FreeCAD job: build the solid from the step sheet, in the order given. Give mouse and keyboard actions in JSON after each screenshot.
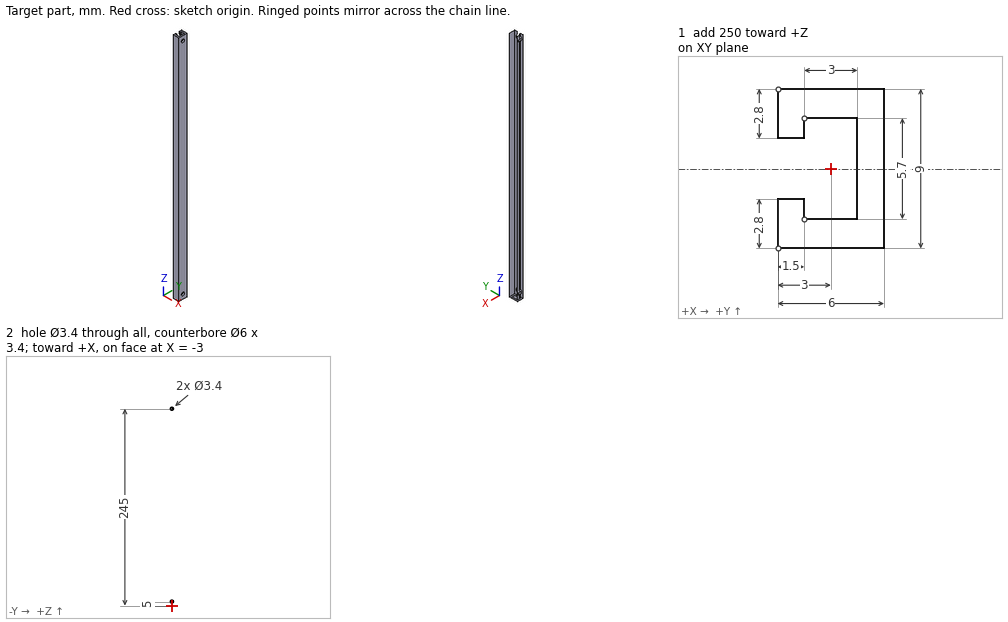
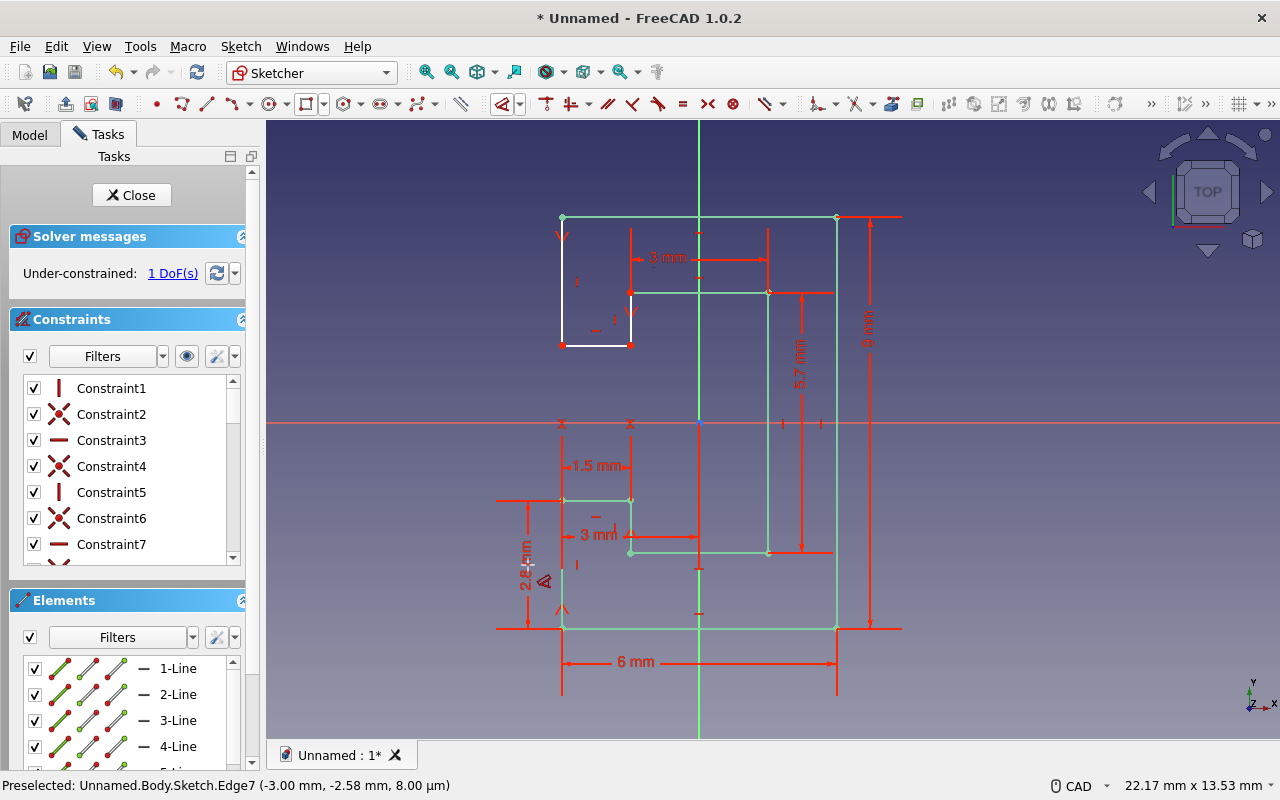
{"action": "left_click", "coordinate": [562, 256]}
{"action": "left_click", "coordinate": [528, 282]}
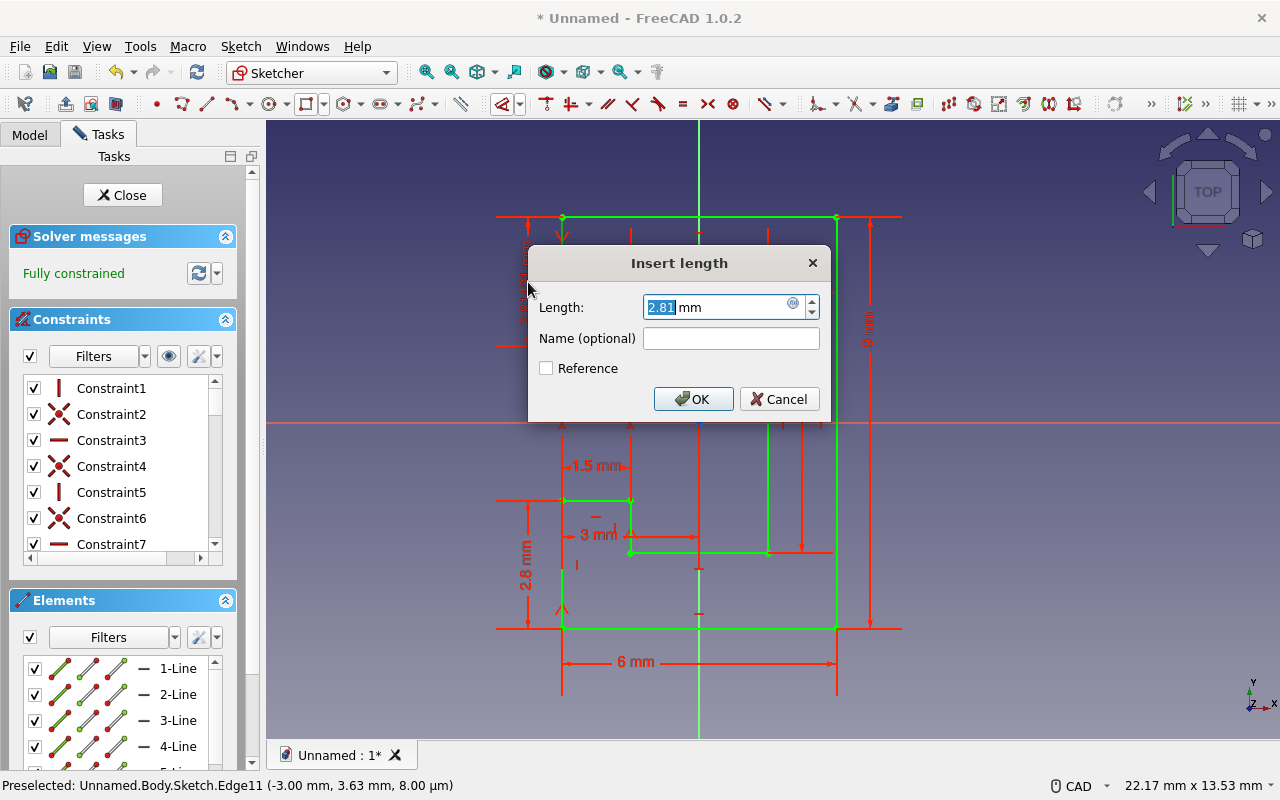
{"action": "type", "text": "2.8"}
{"action": "key", "text": "Return"}
{"action": "key", "text": "Escape"}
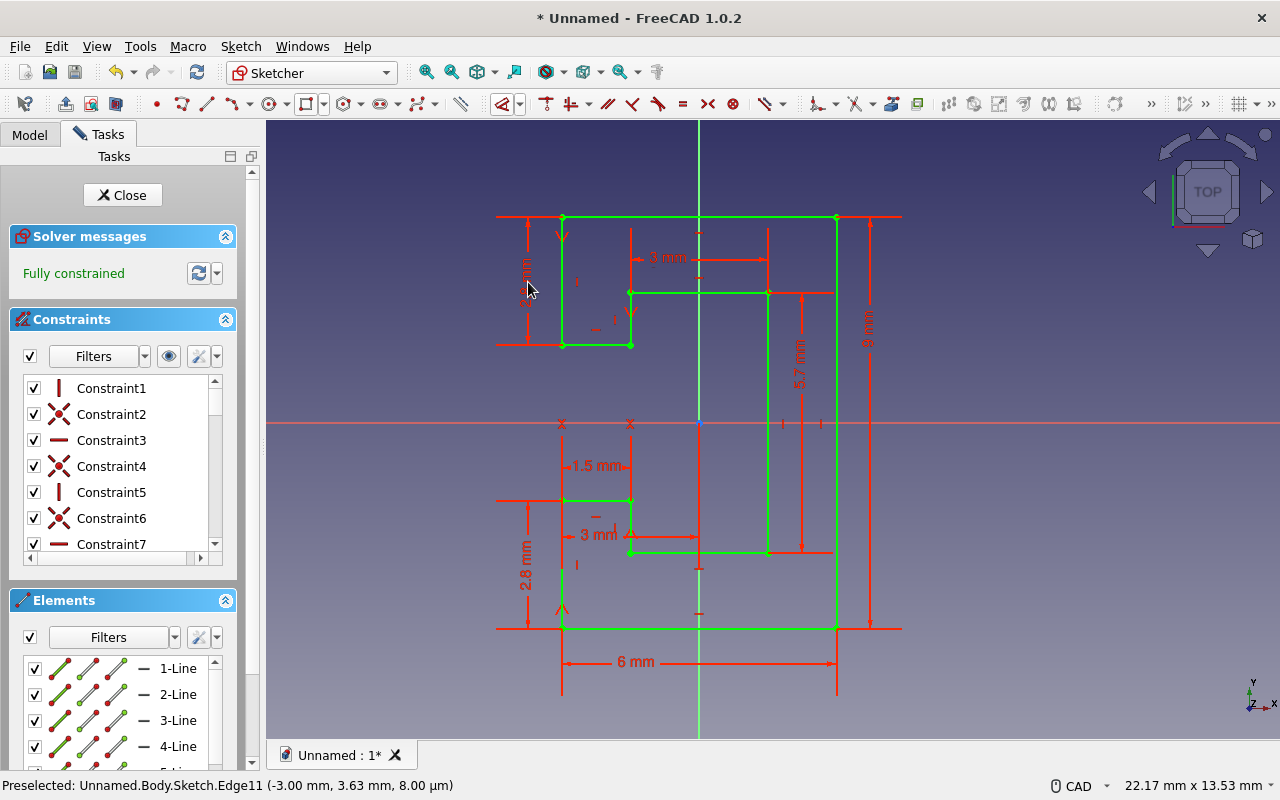
{"action": "left_click", "coordinate": [123, 195]}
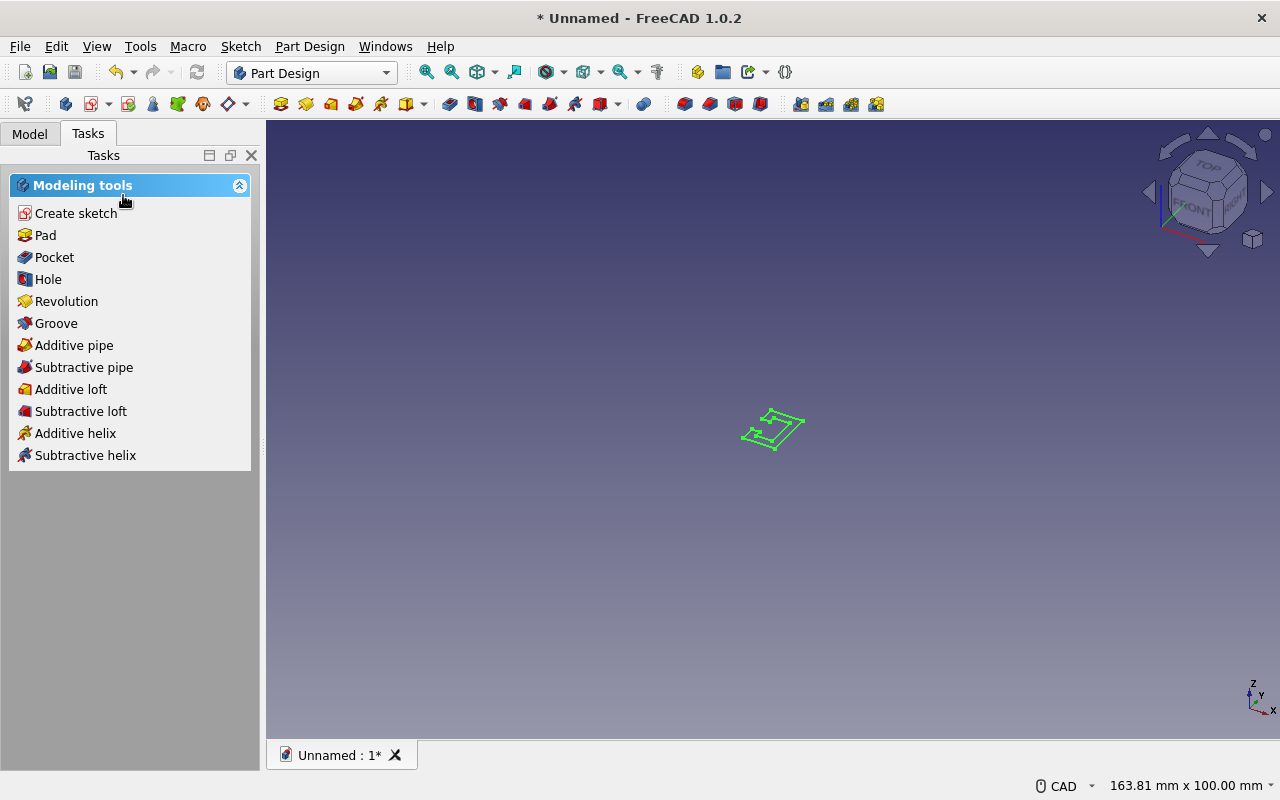
{"action": "left_click", "coordinate": [281, 104]}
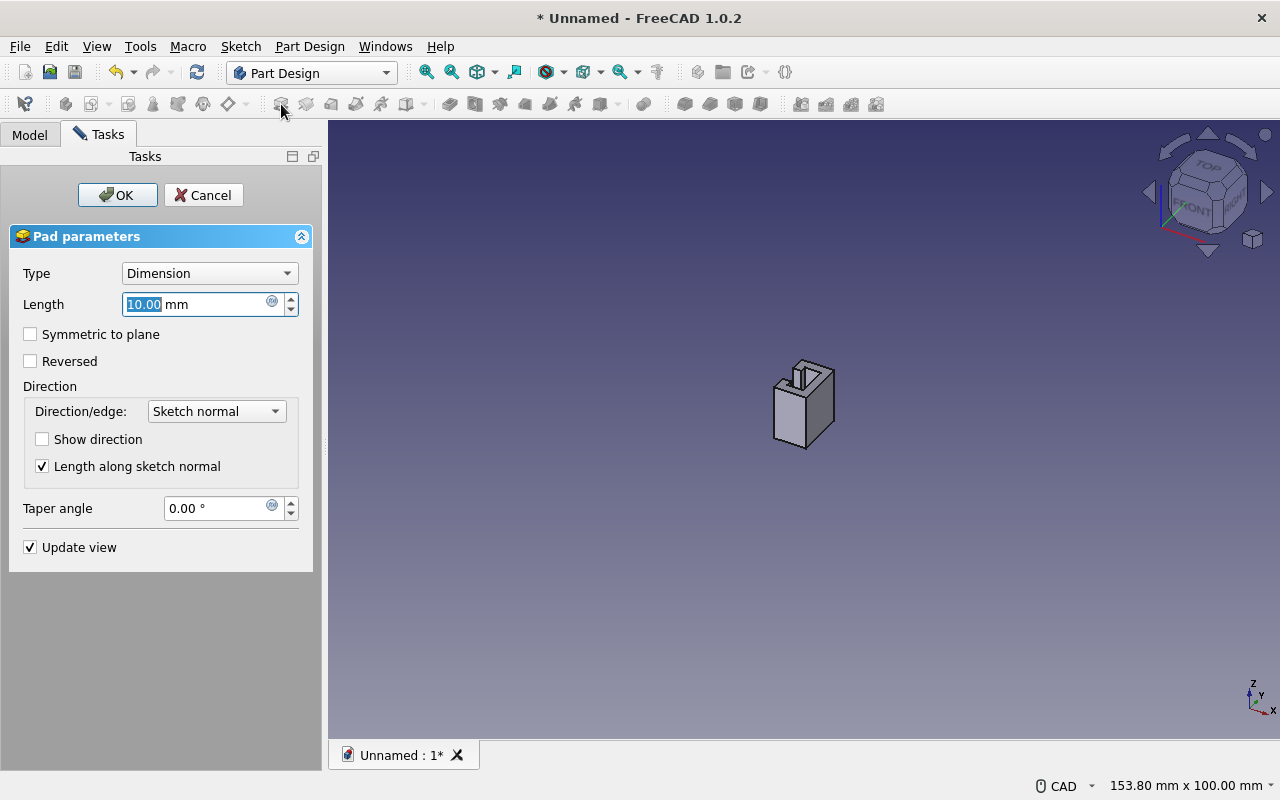
{"action": "type", "text": "250"}
{"action": "key", "text": "Tab"}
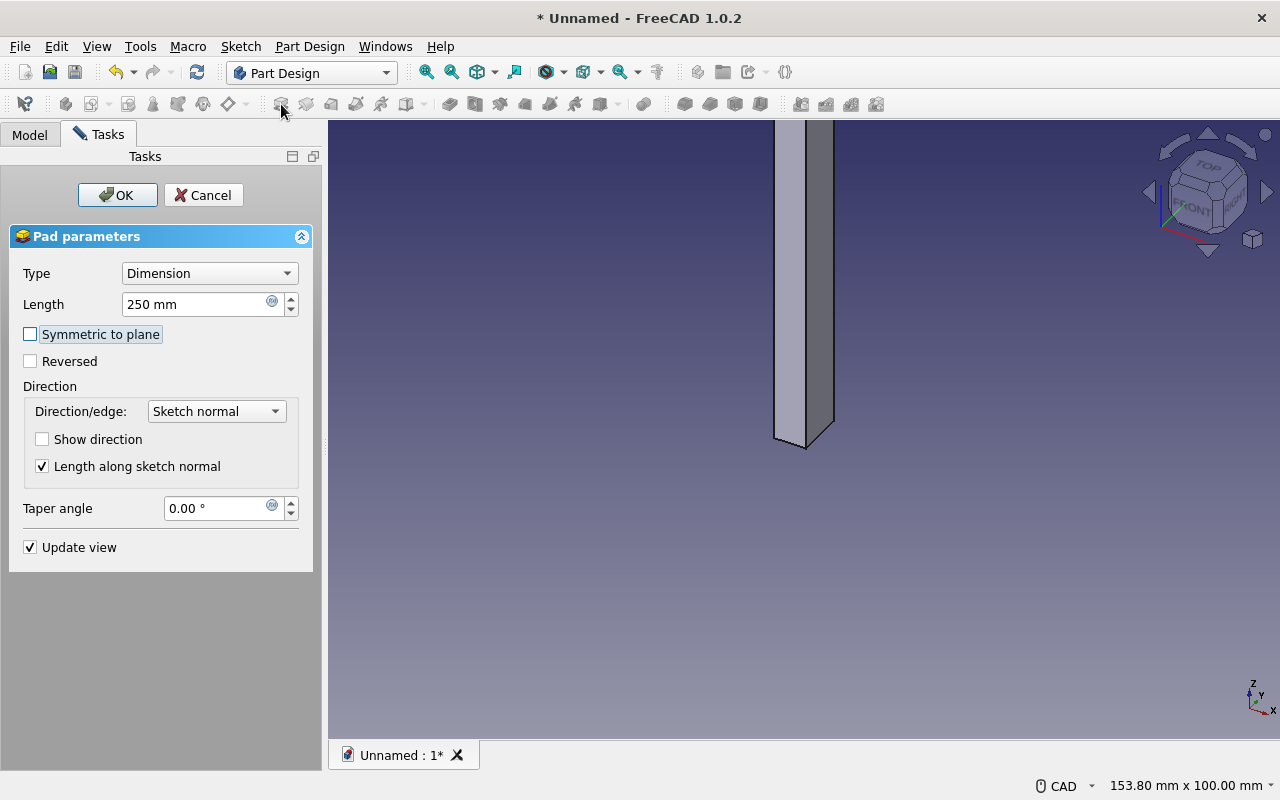
{"action": "left_click", "coordinate": [118, 195]}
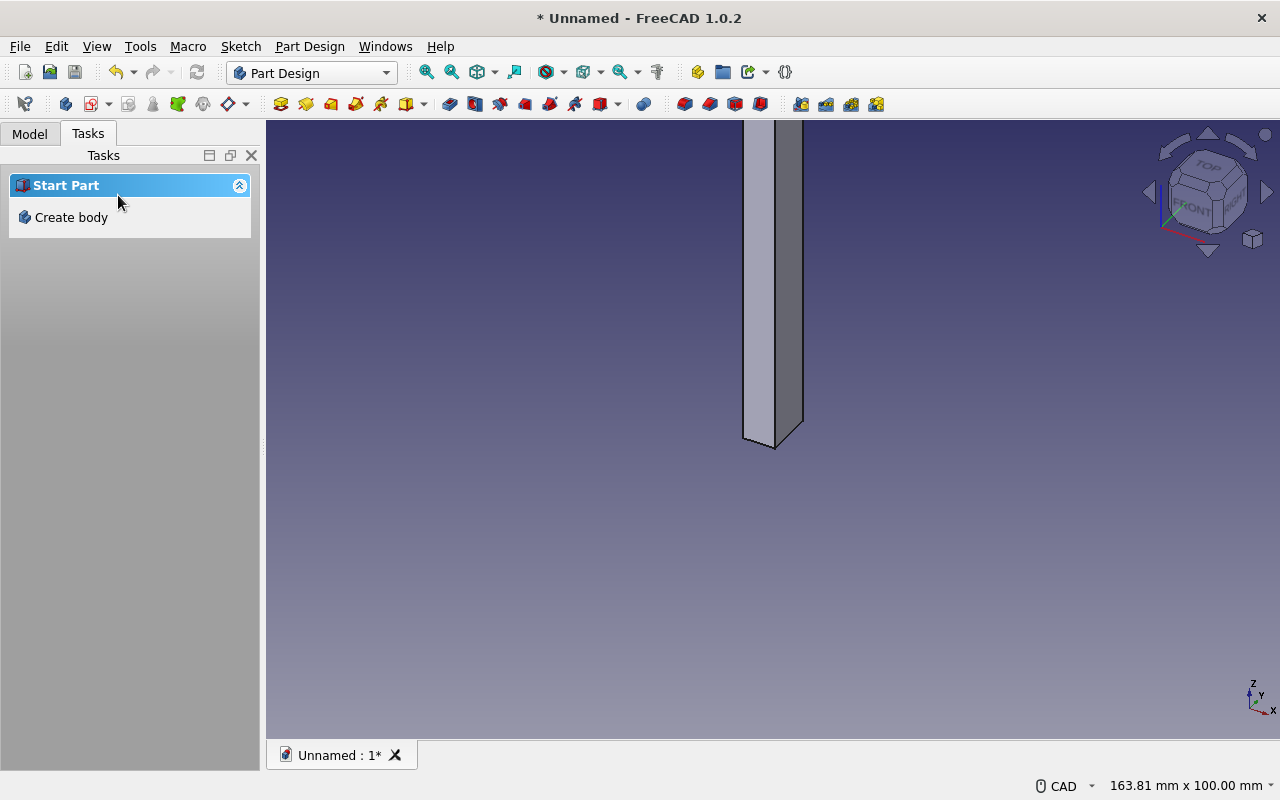
{"action": "key", "text": "v f"}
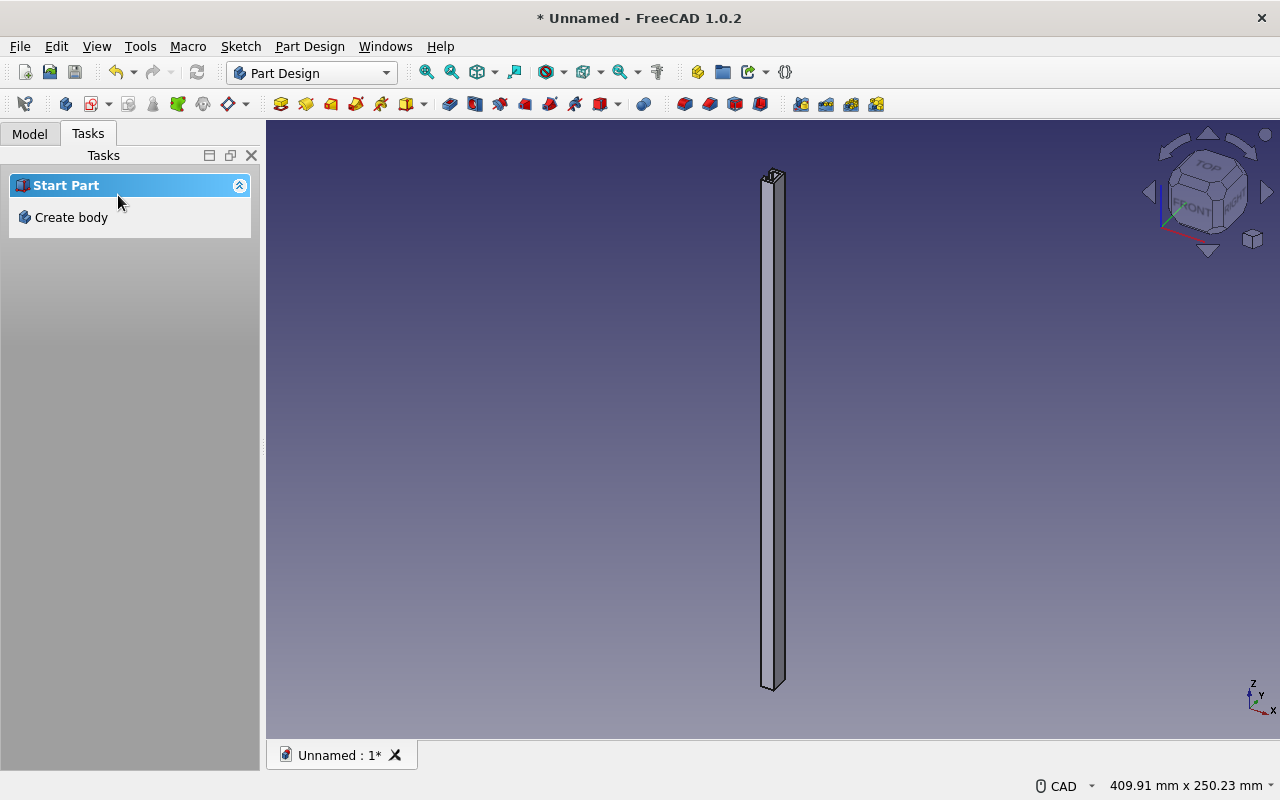
{"action": "key", "text": "6"}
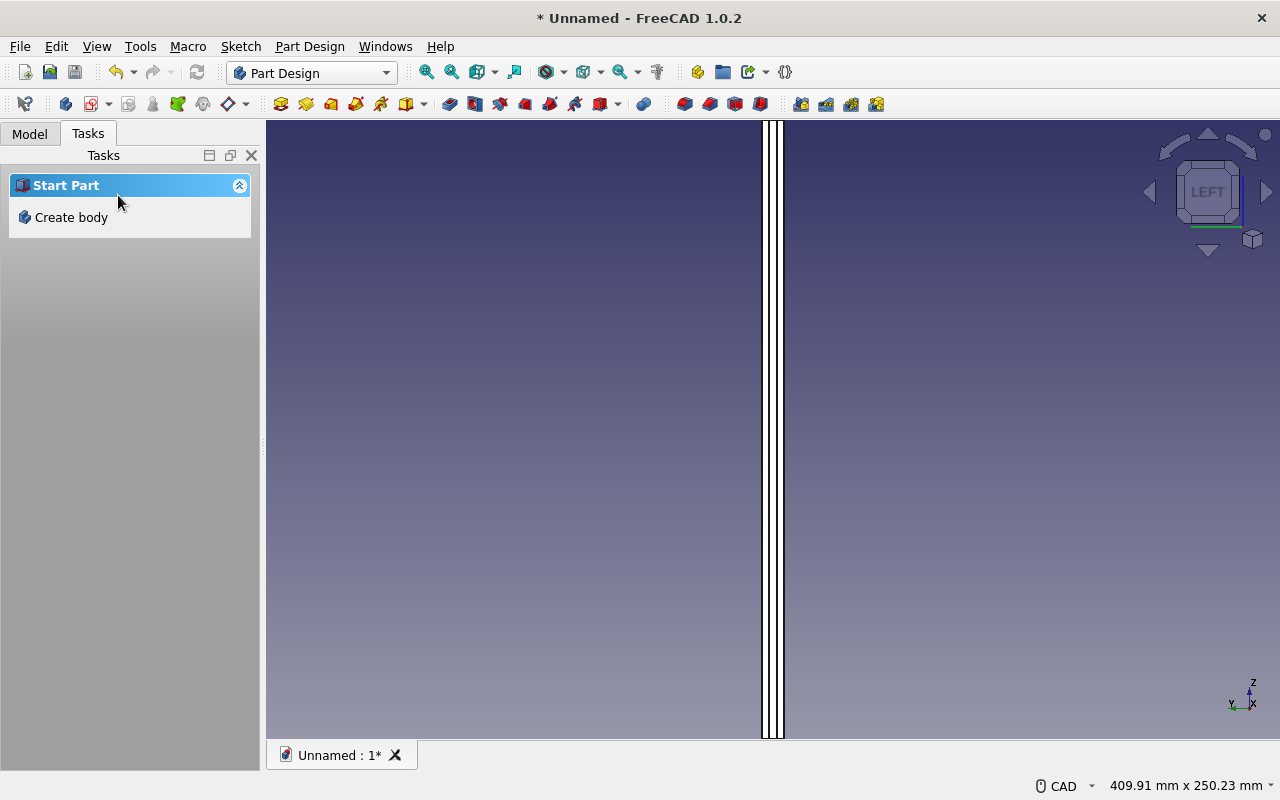
{"action": "left_click", "coordinate": [427, 72]}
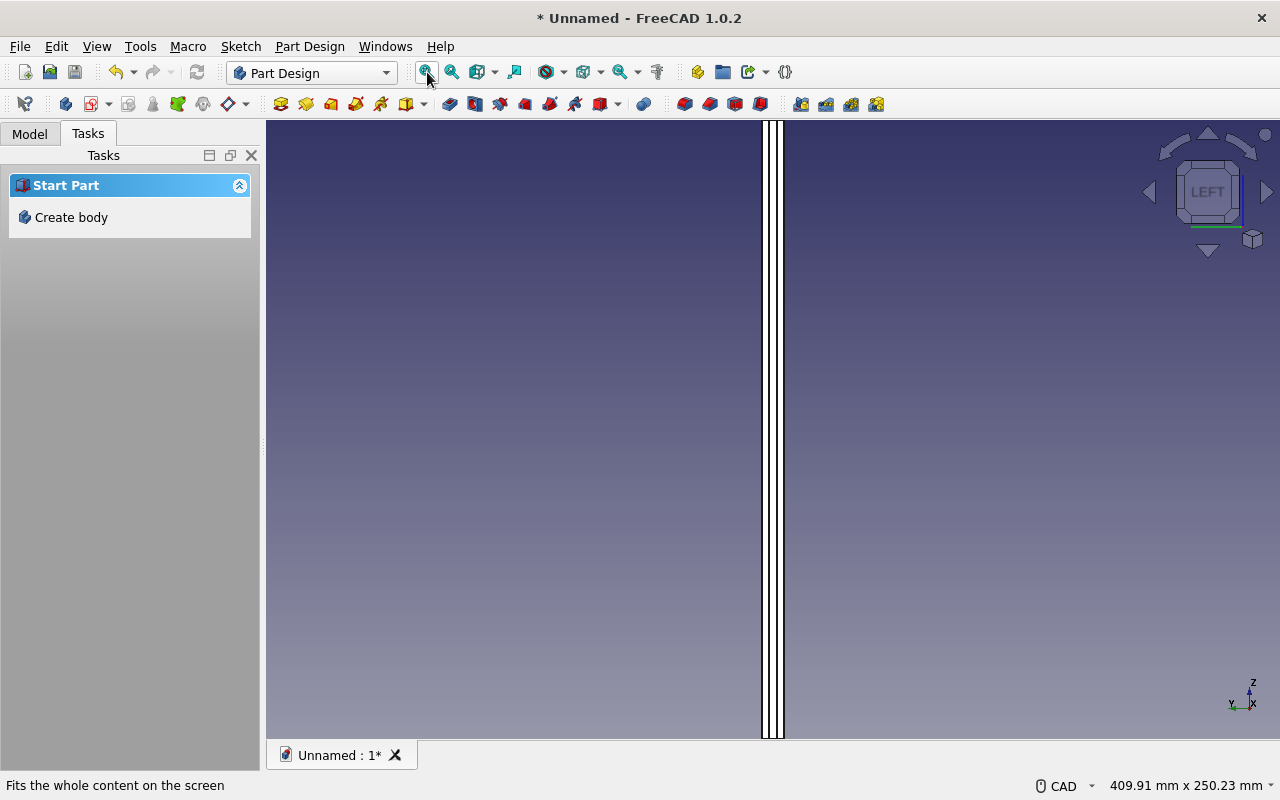
{"action": "scroll", "coordinate": [781, 163], "scroll_direction": "up", "scroll_amount": 7}